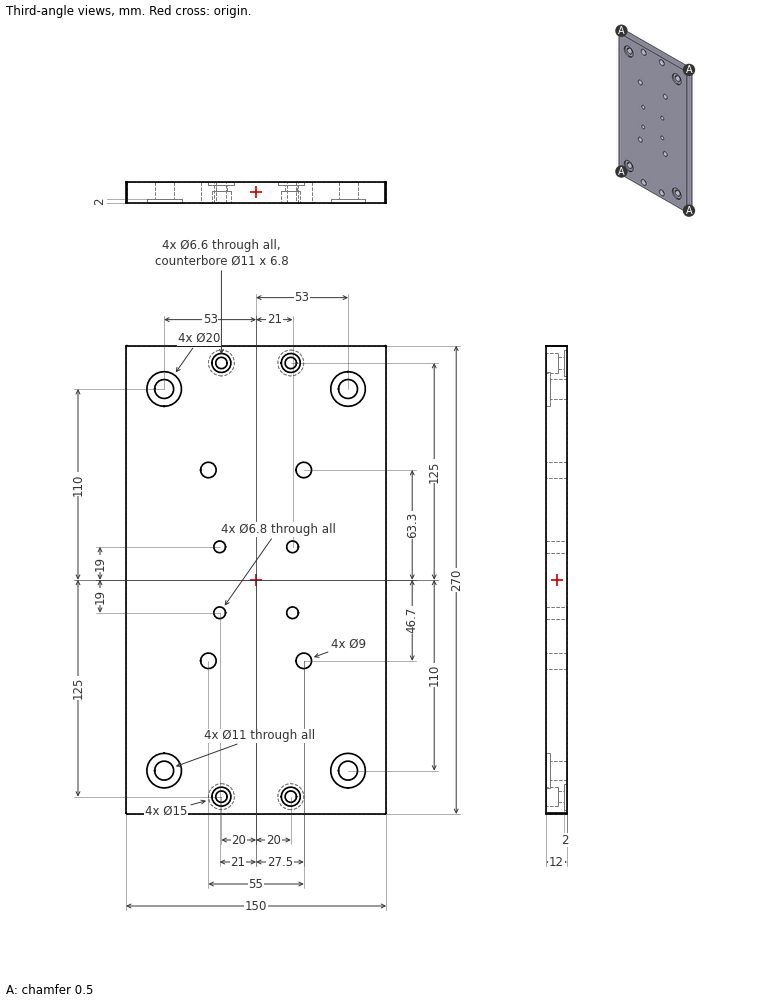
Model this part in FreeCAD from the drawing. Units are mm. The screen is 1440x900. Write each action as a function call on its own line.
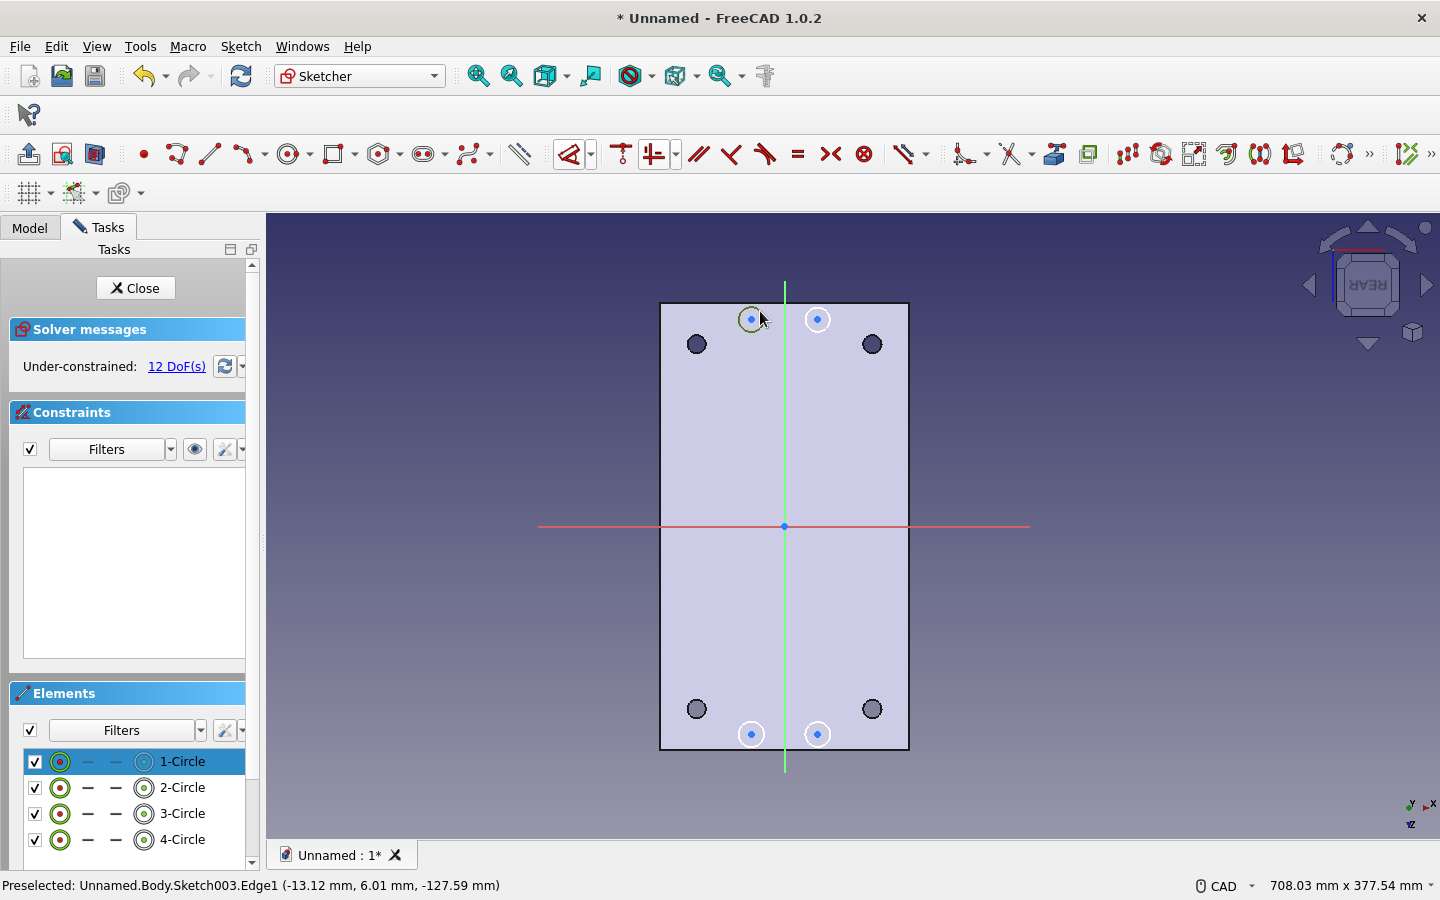
click(826, 311)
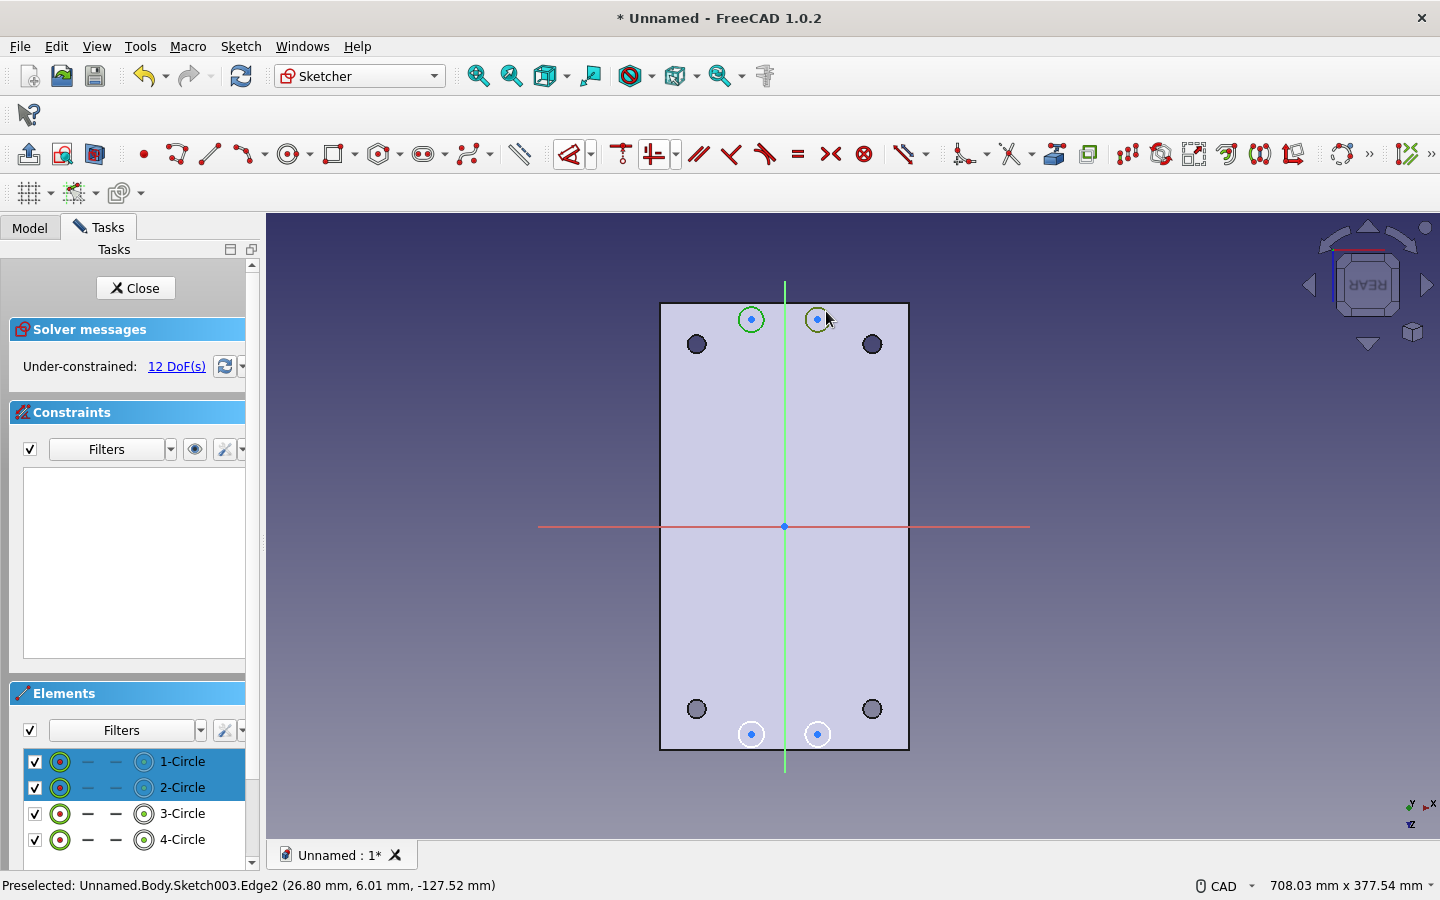
click(827, 726)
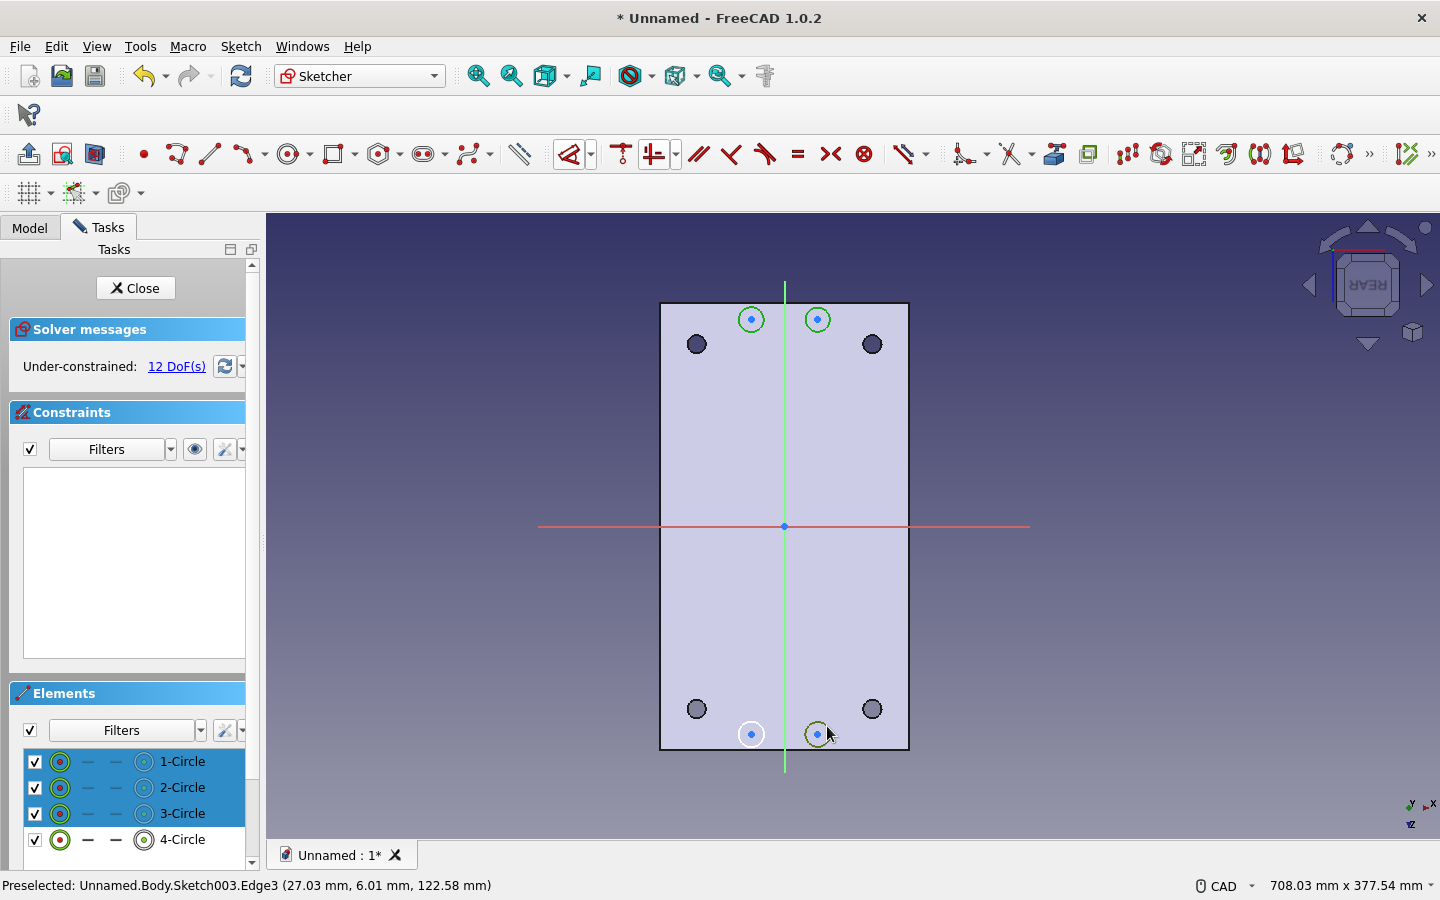
click(760, 725)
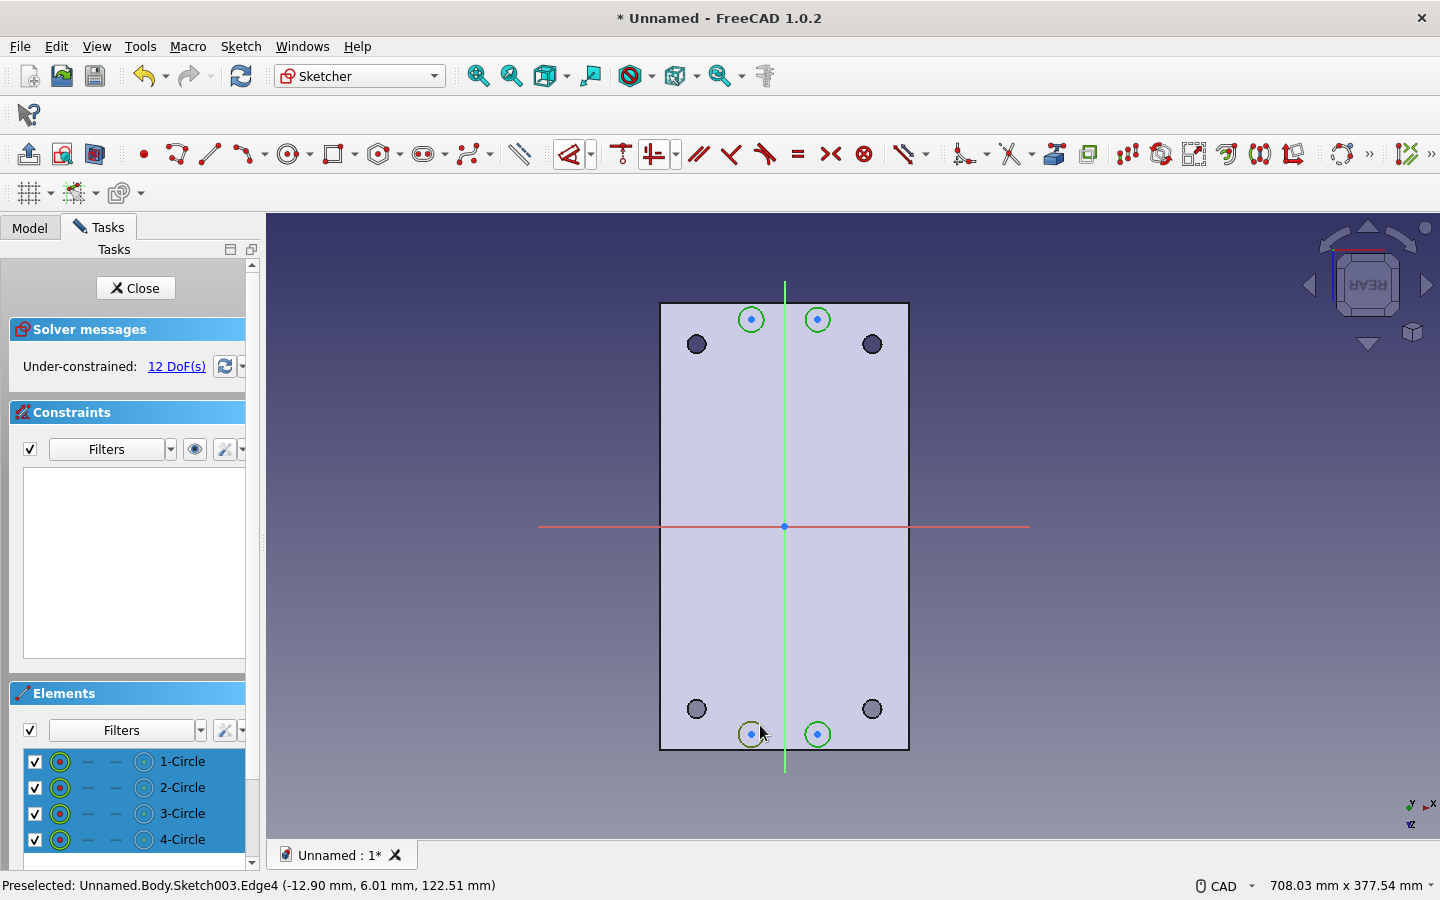
click(798, 154)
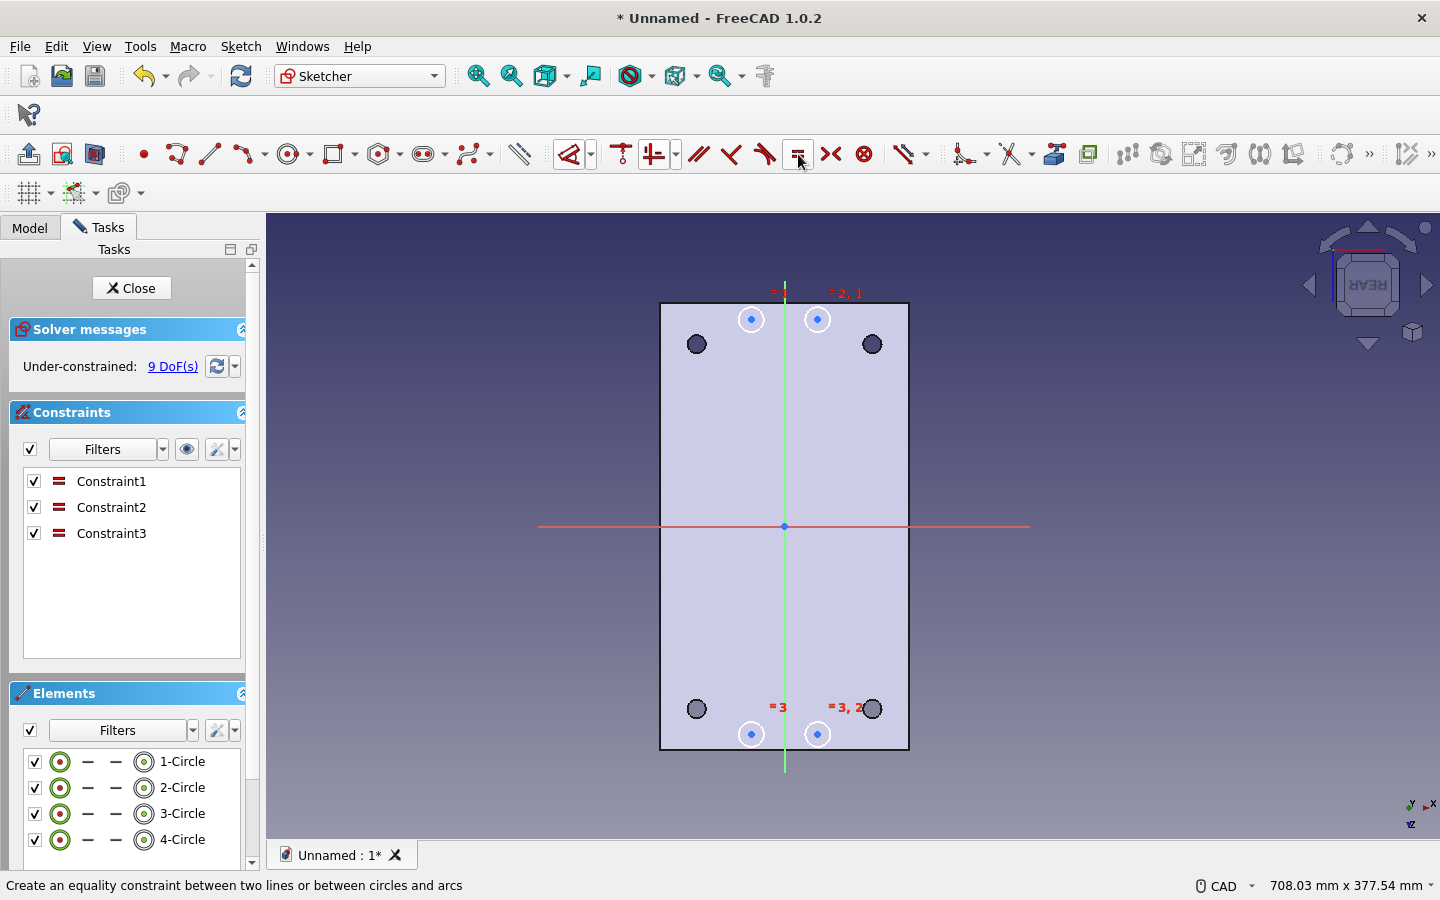
click(751, 320)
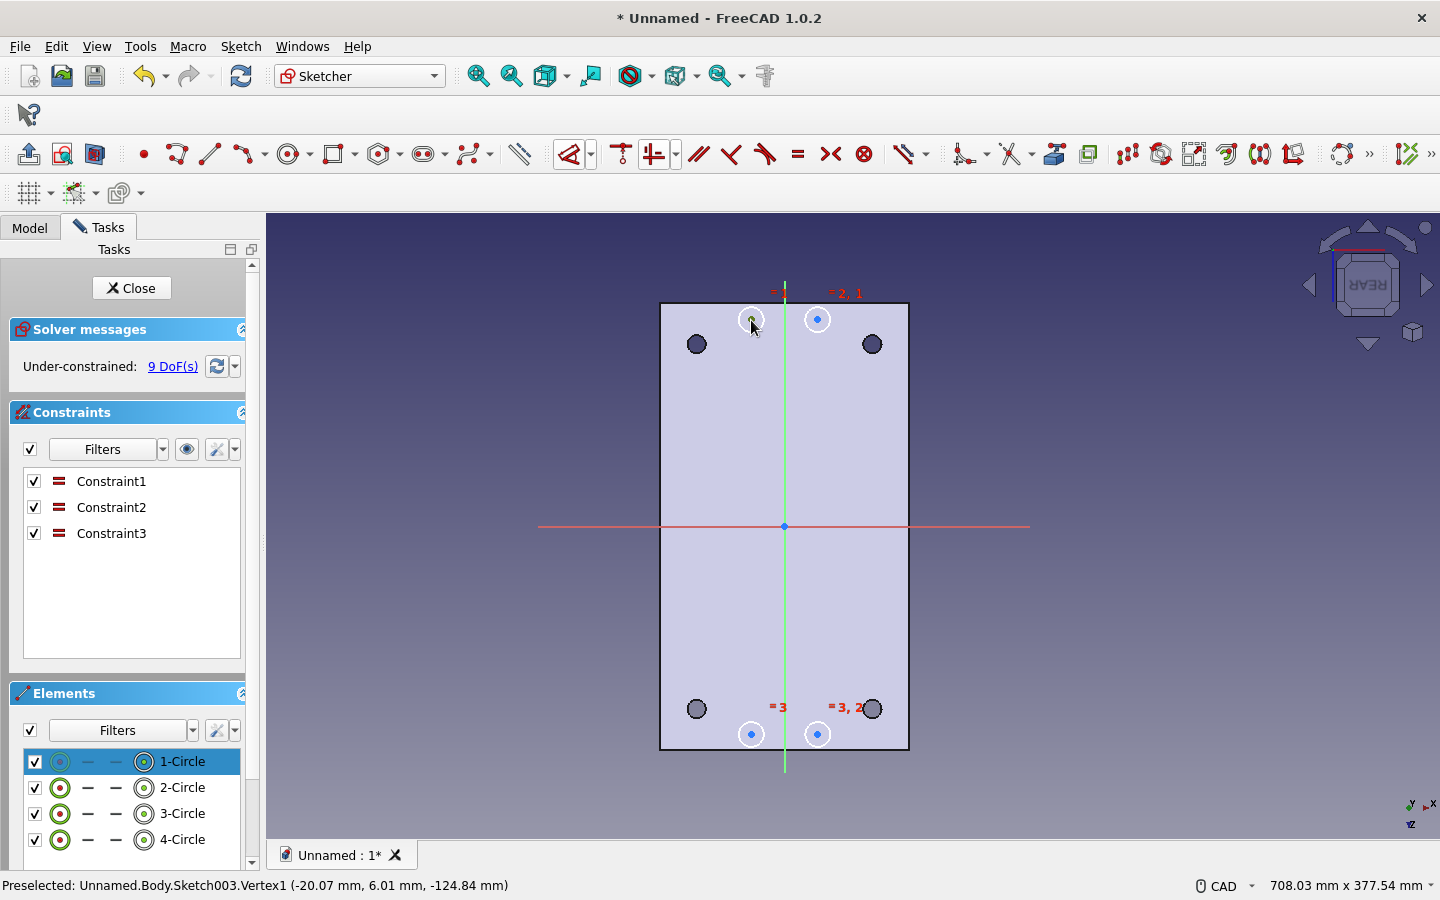
click(818, 320)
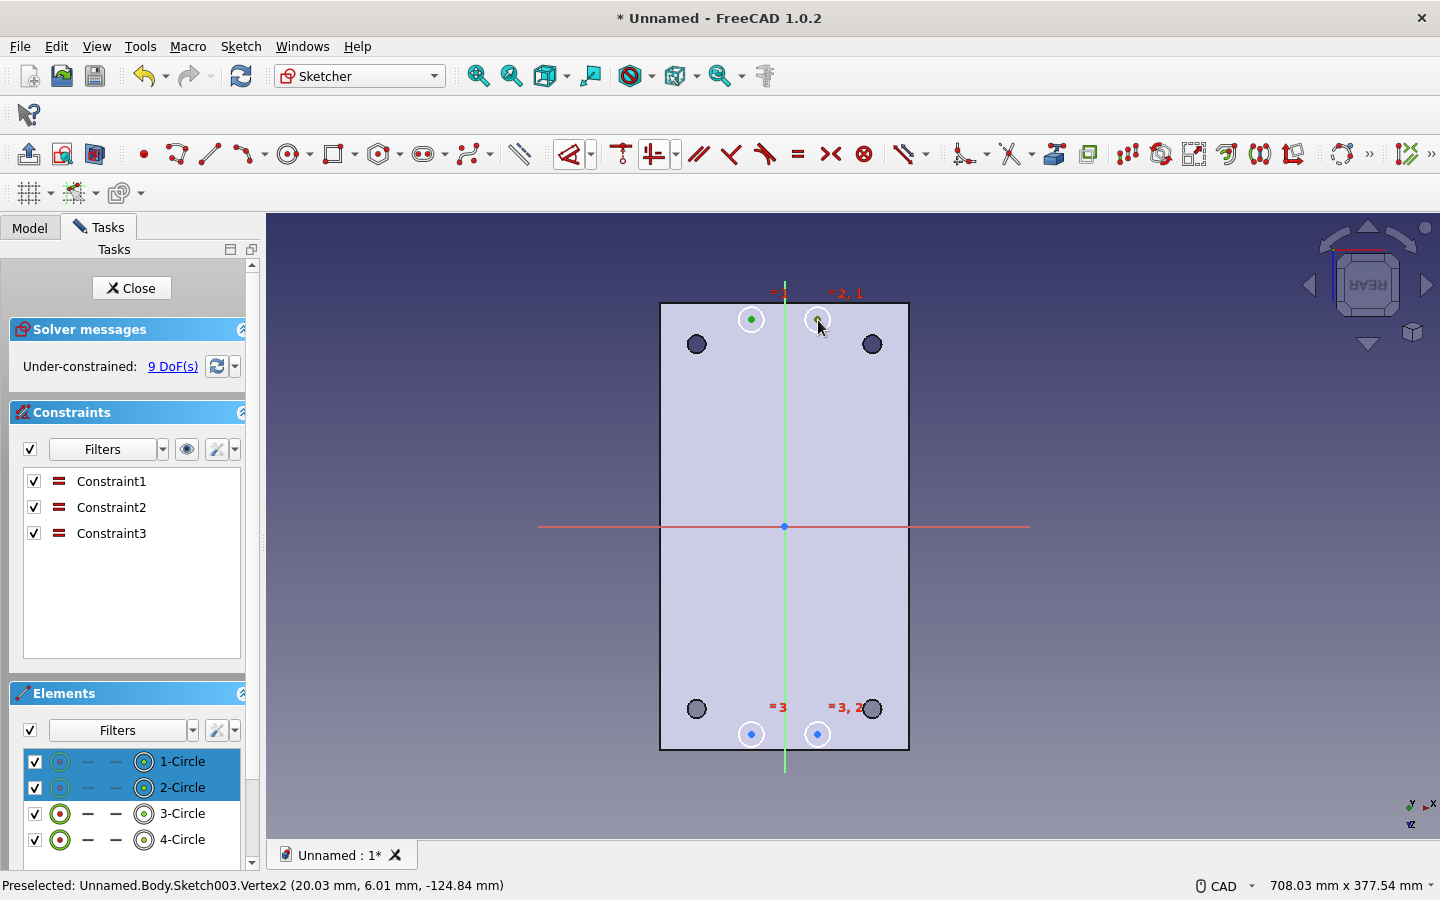
key(h)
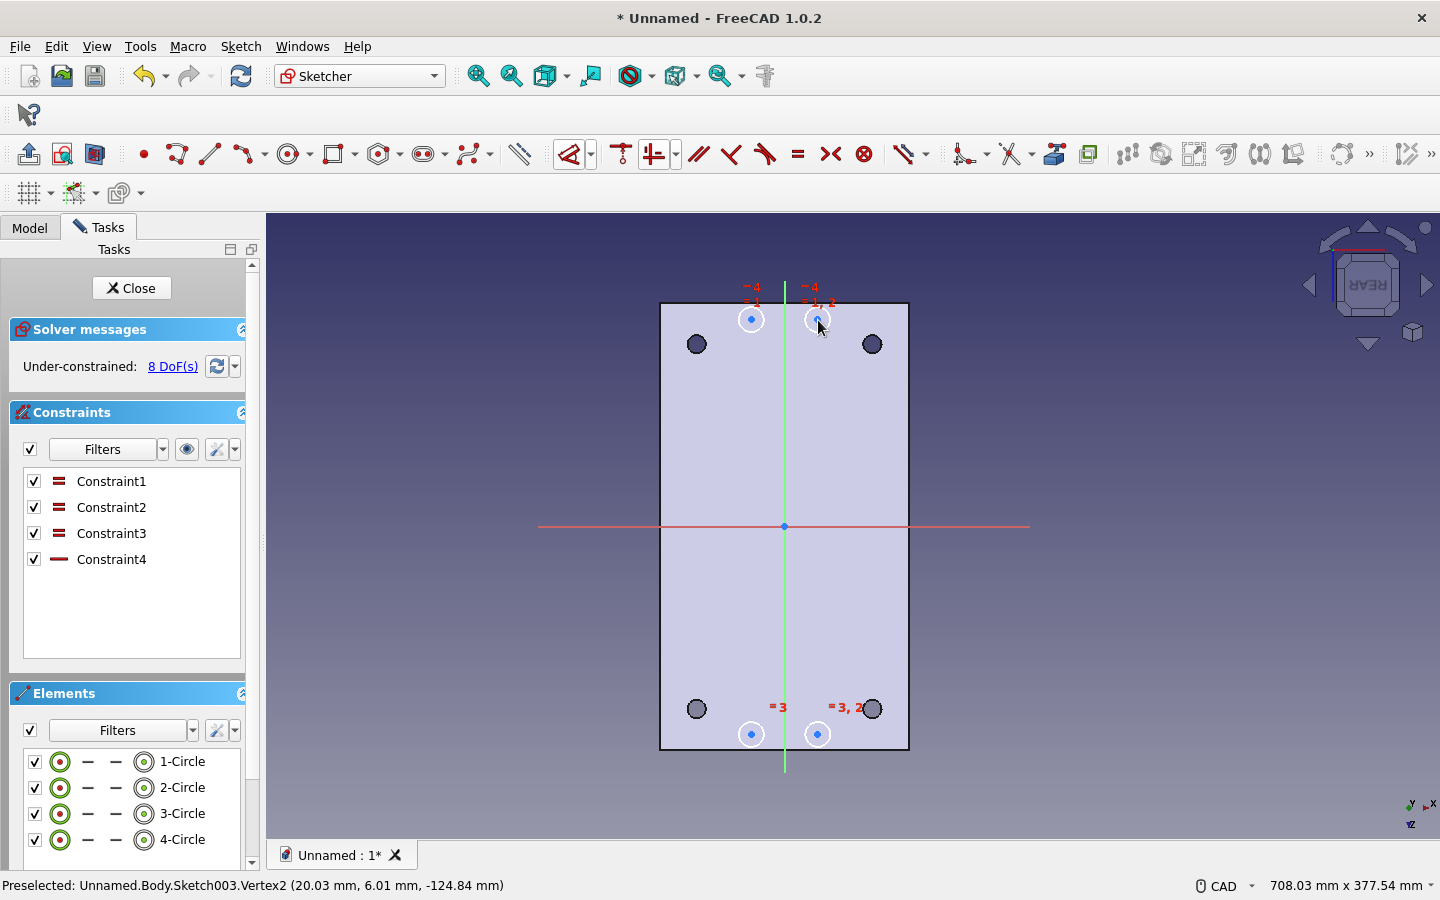
click(818, 320)